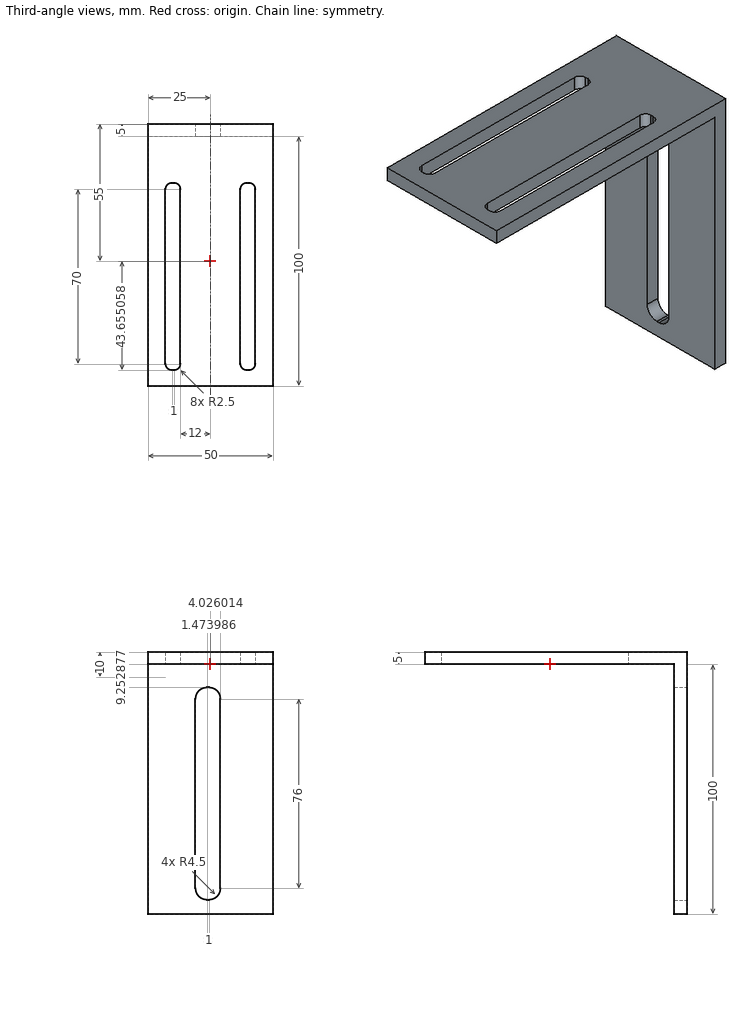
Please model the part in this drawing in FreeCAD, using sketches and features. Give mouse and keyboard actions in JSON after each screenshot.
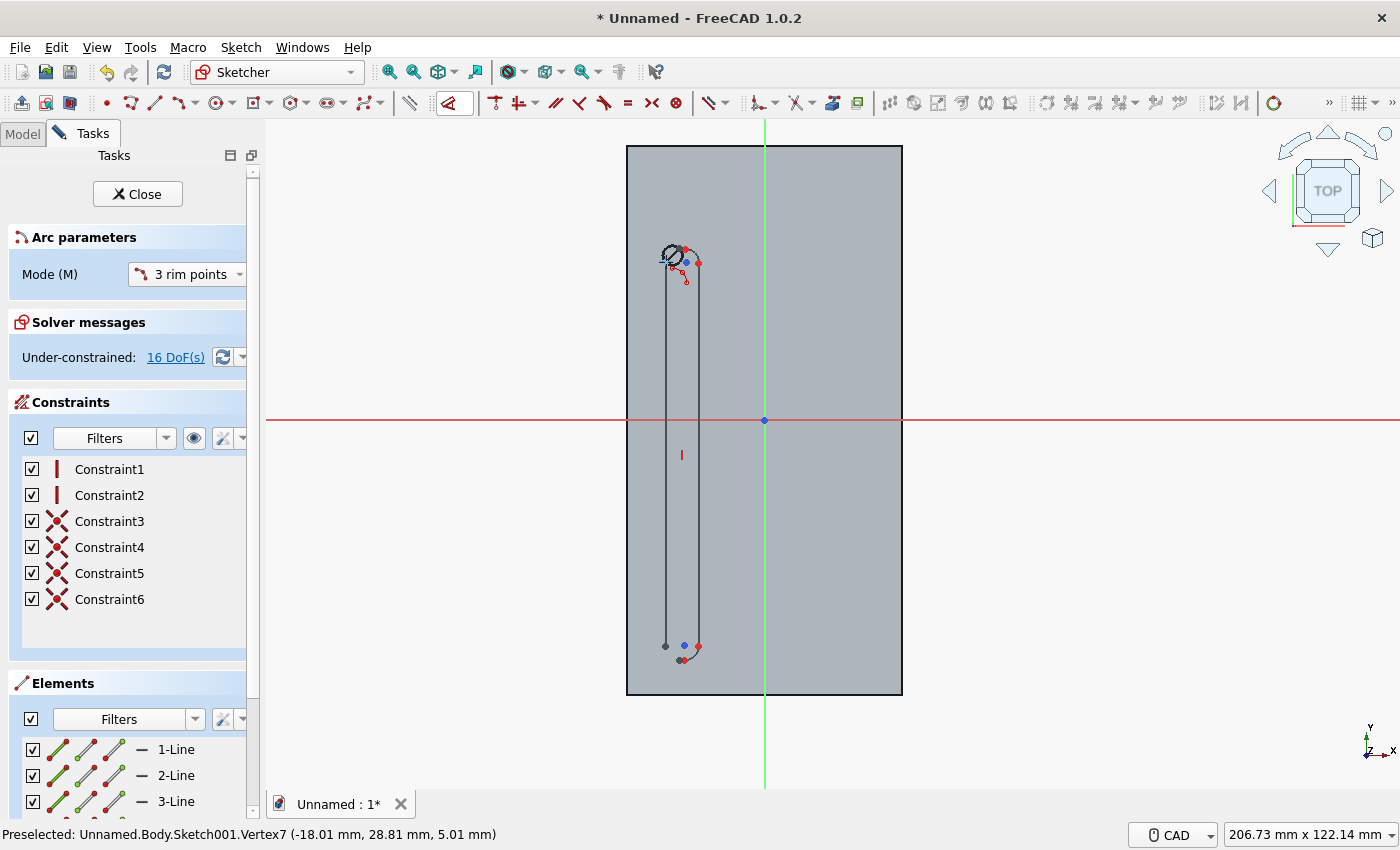
{"action": "scroll", "coordinate": [670, 252], "scroll_direction": "up", "scroll_amount": 7}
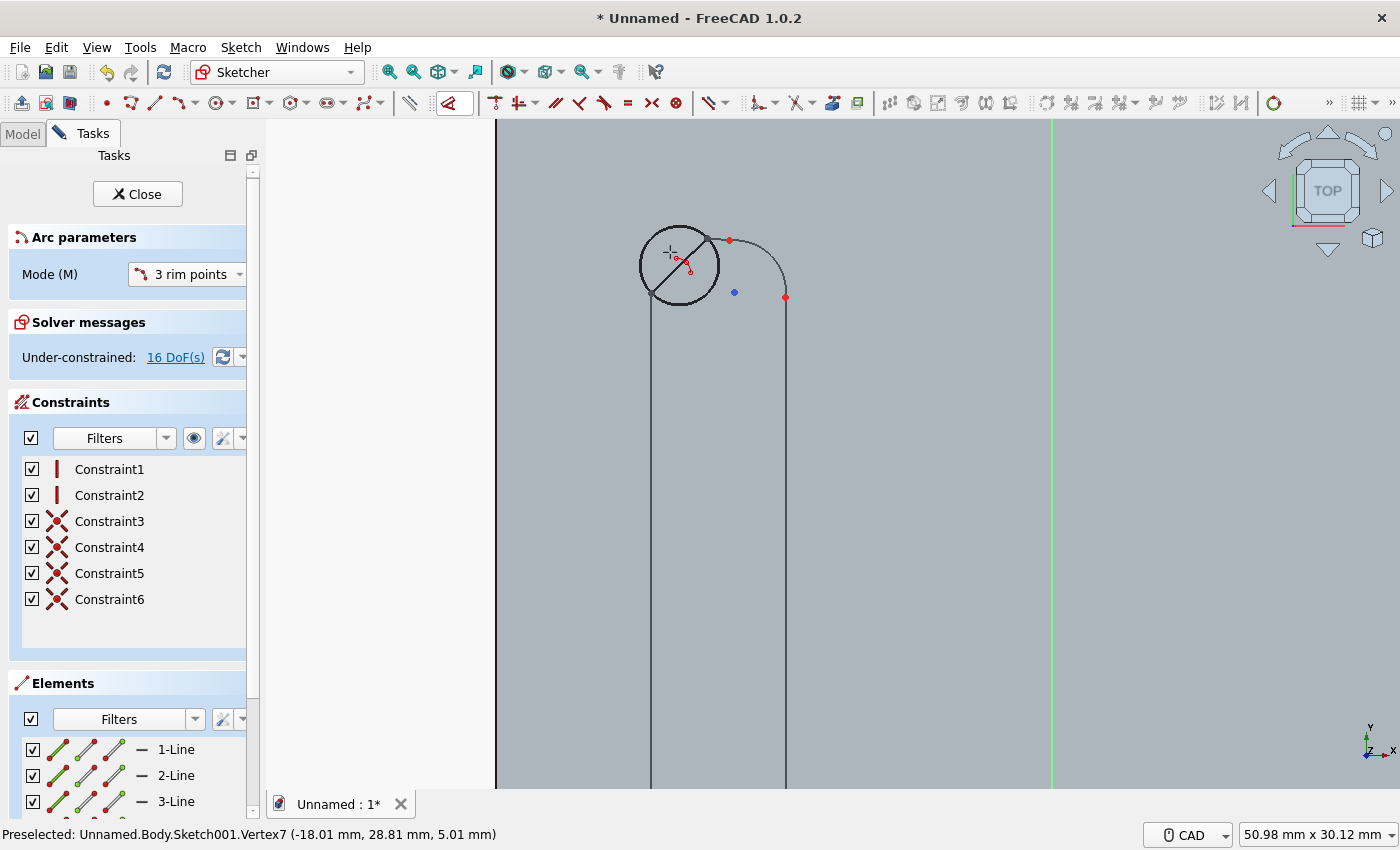
{"action": "left_click", "coordinate": [668, 253]}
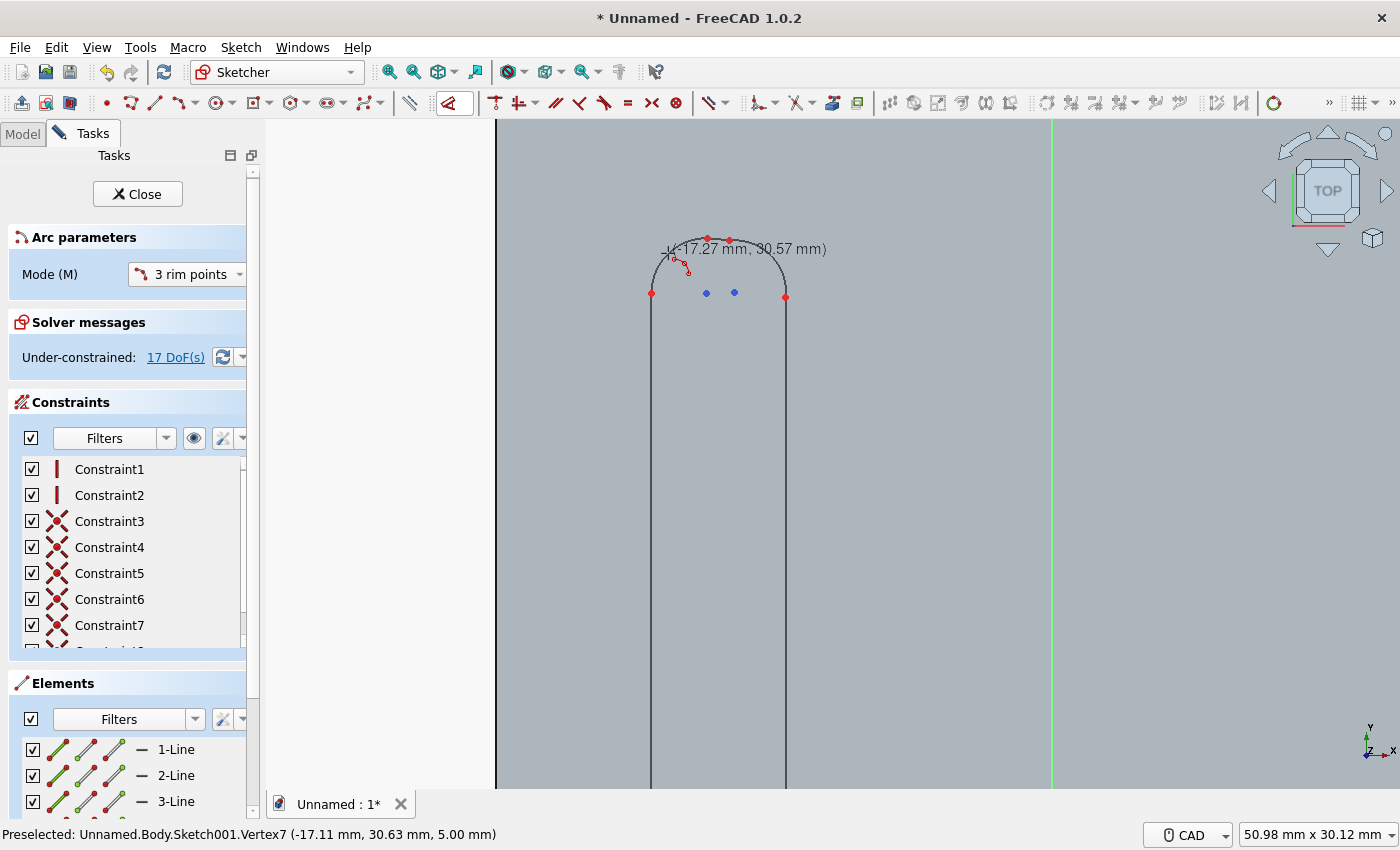
{"action": "scroll", "coordinate": [670, 252], "scroll_direction": "down", "scroll_amount": 7}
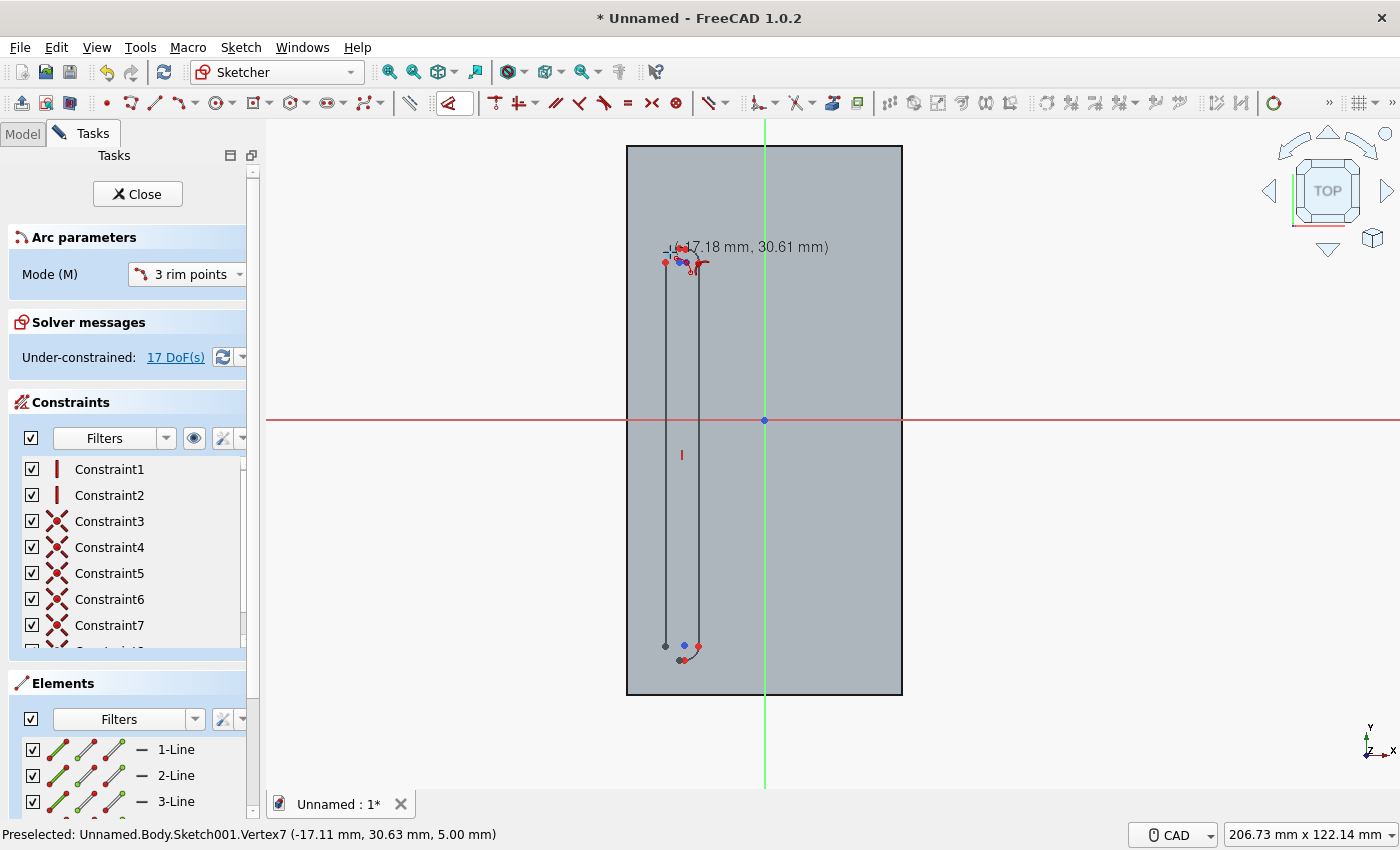
{"action": "left_click", "coordinate": [666, 647]}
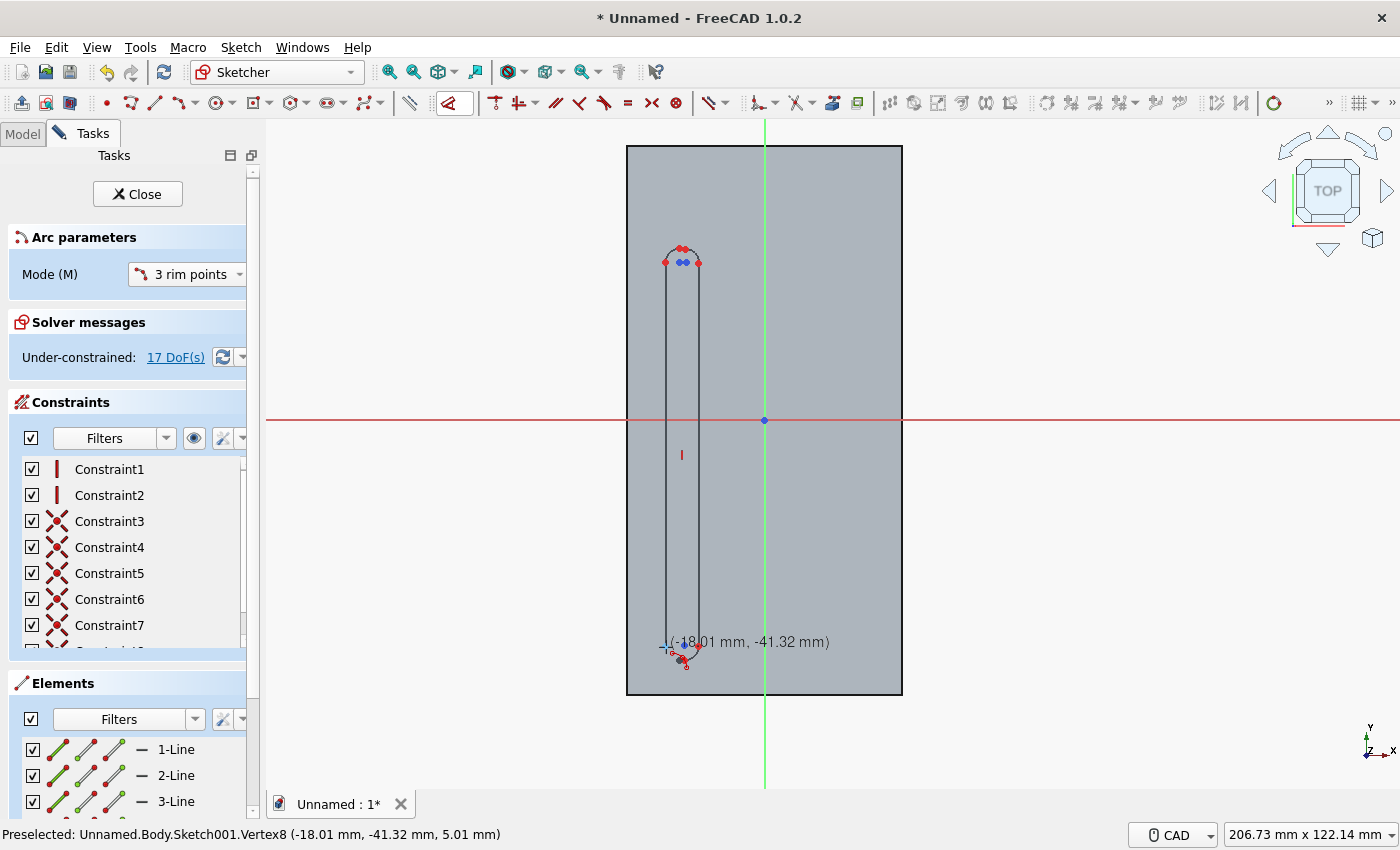
{"action": "scroll", "coordinate": [679, 660], "scroll_direction": "up", "scroll_amount": 9}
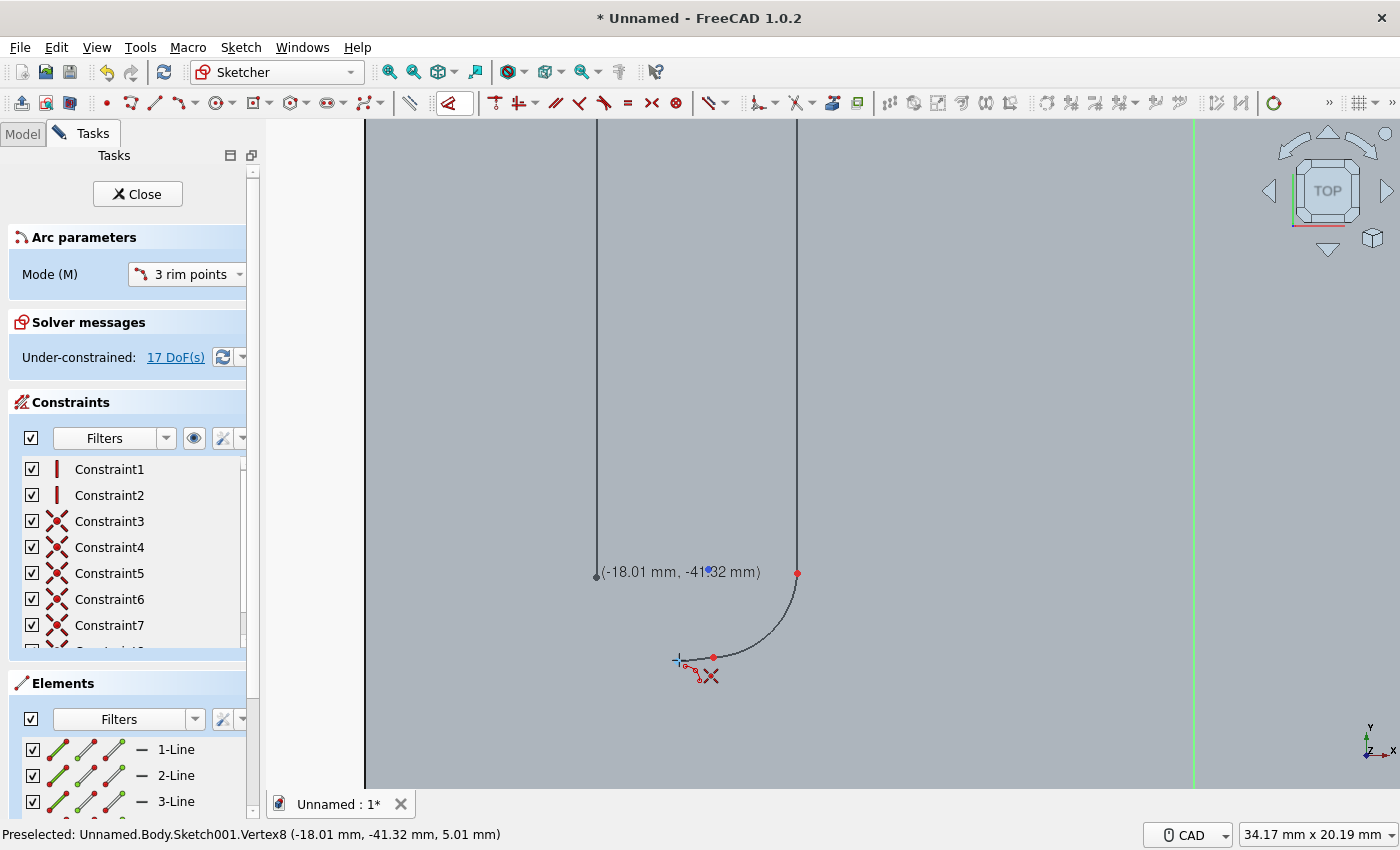
{"action": "left_click", "coordinate": [677, 662]}
{"action": "left_click", "coordinate": [621, 630]}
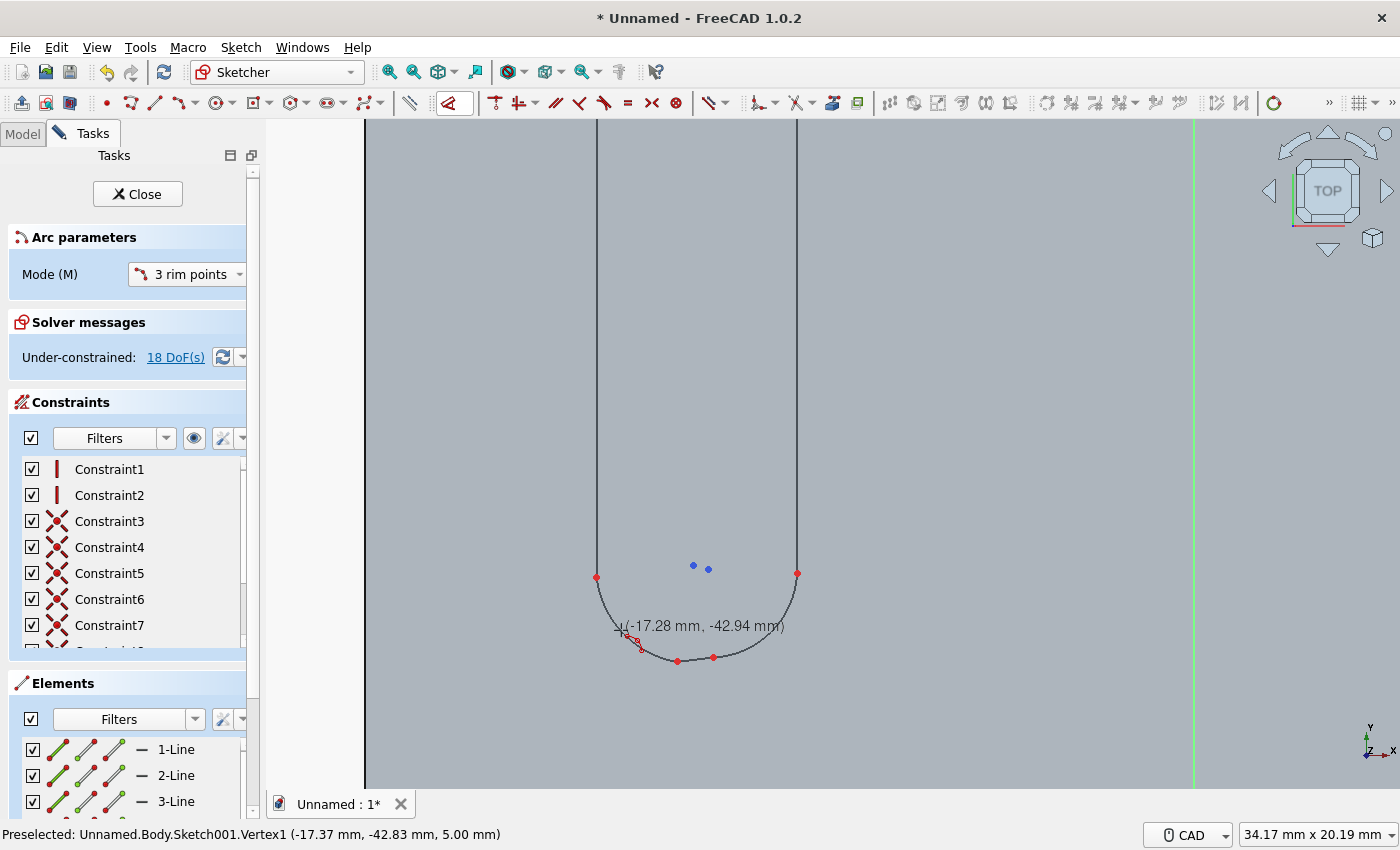
{"action": "key", "text": "g l"}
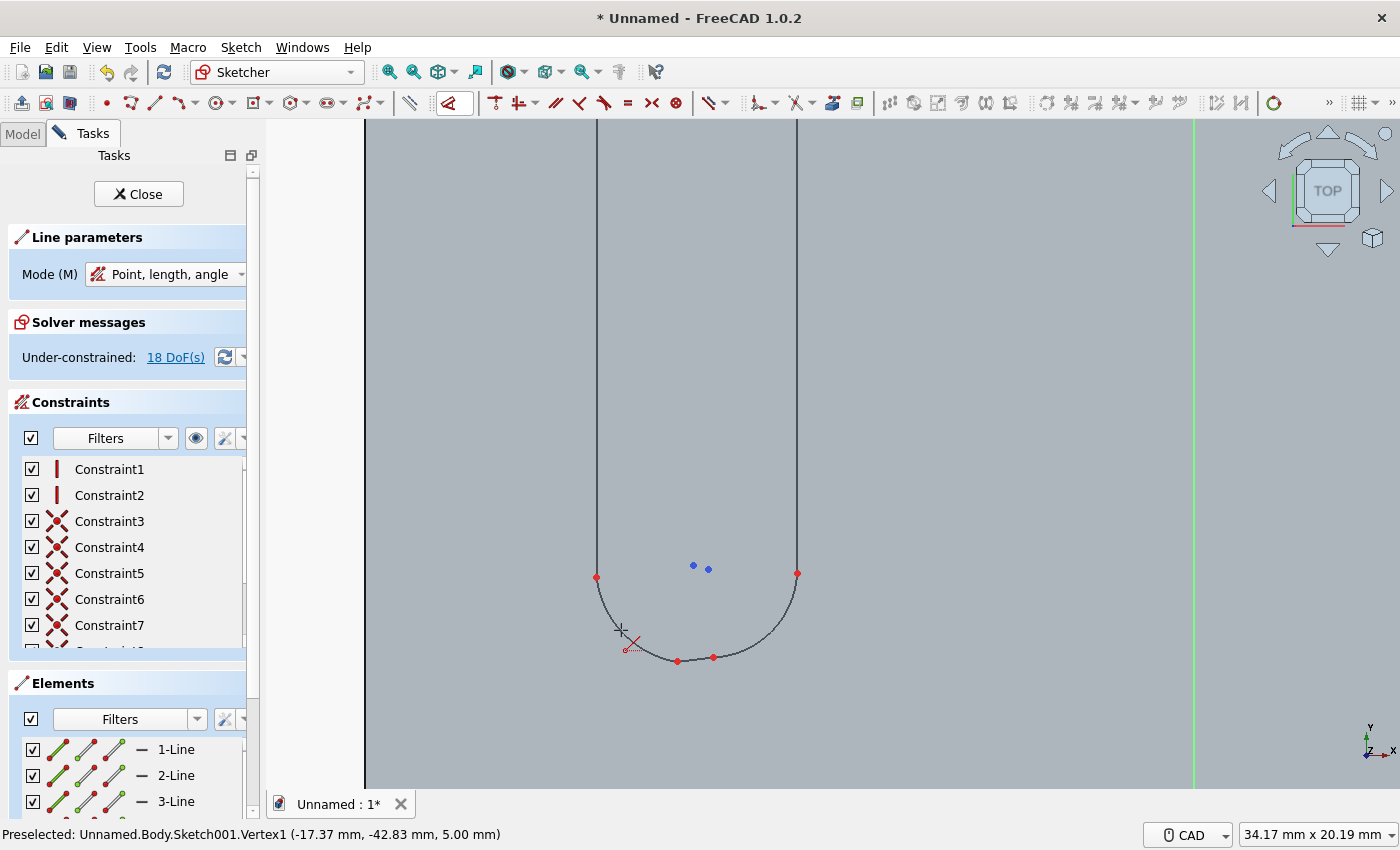
{"action": "scroll", "coordinate": [679, 661], "scroll_direction": "down", "scroll_amount": 9}